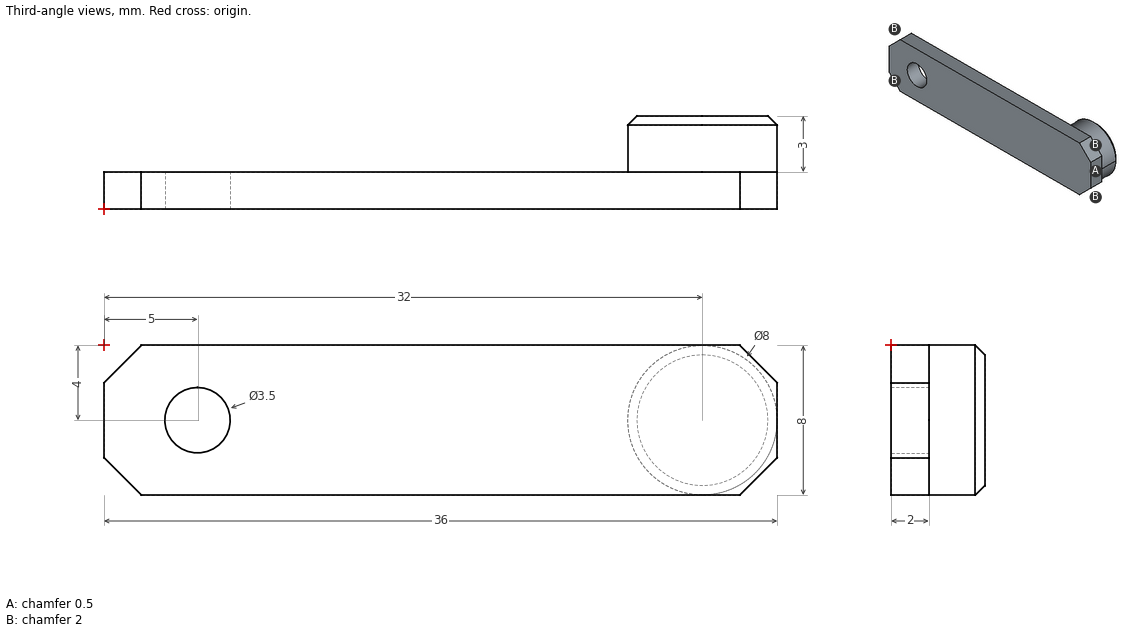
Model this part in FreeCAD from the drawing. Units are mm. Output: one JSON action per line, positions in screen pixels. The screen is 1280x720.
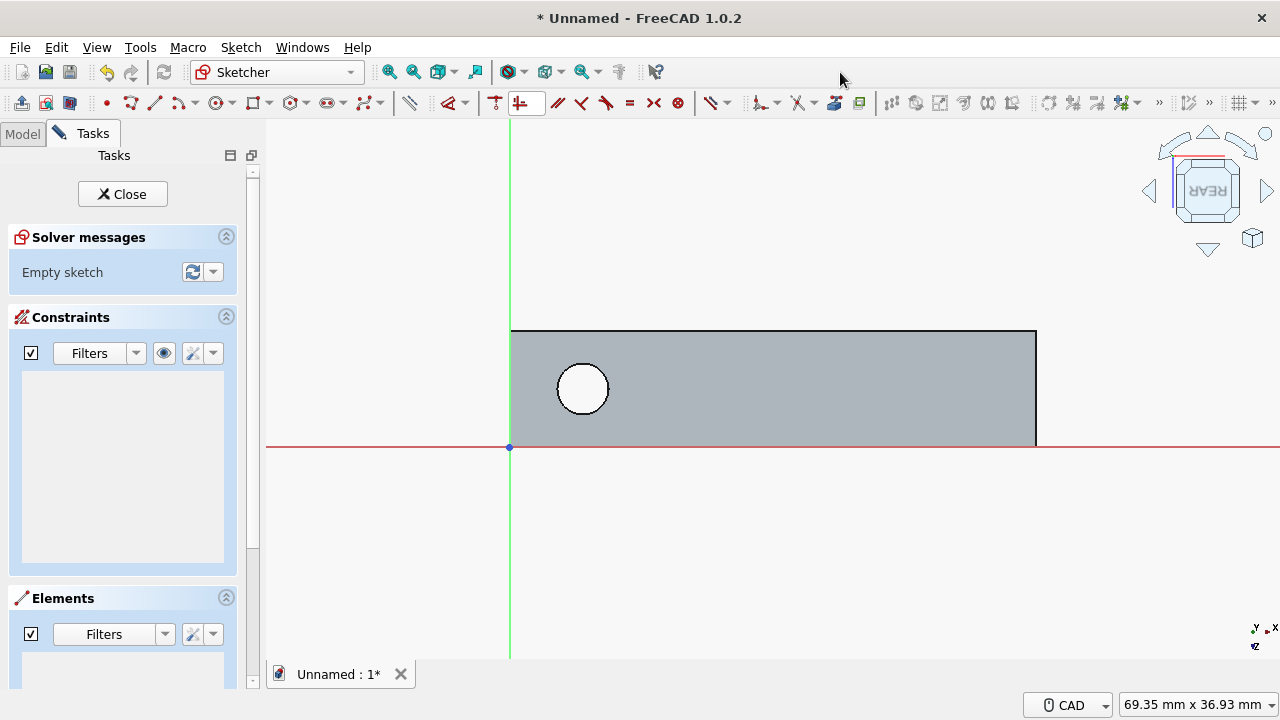
{"action": "scroll", "coordinate": [1115, 389], "scroll_direction": "up", "scroll_amount": 5}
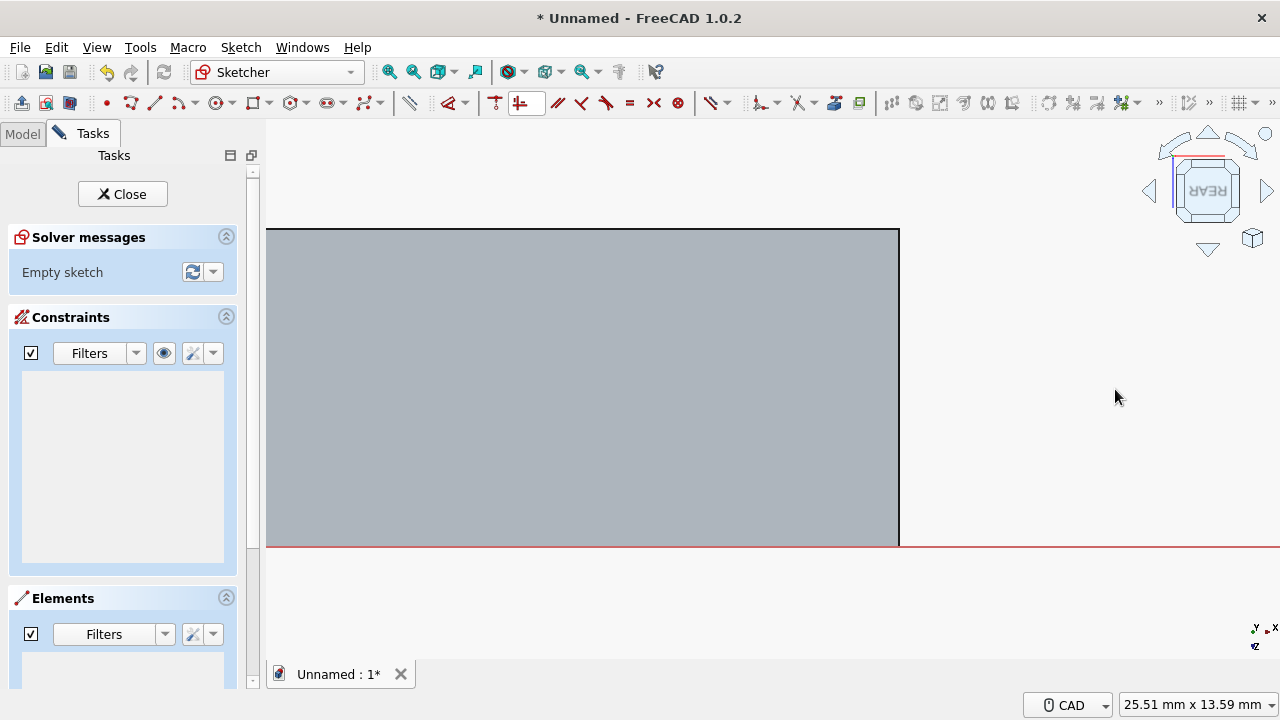
{"action": "key", "text": "g c"}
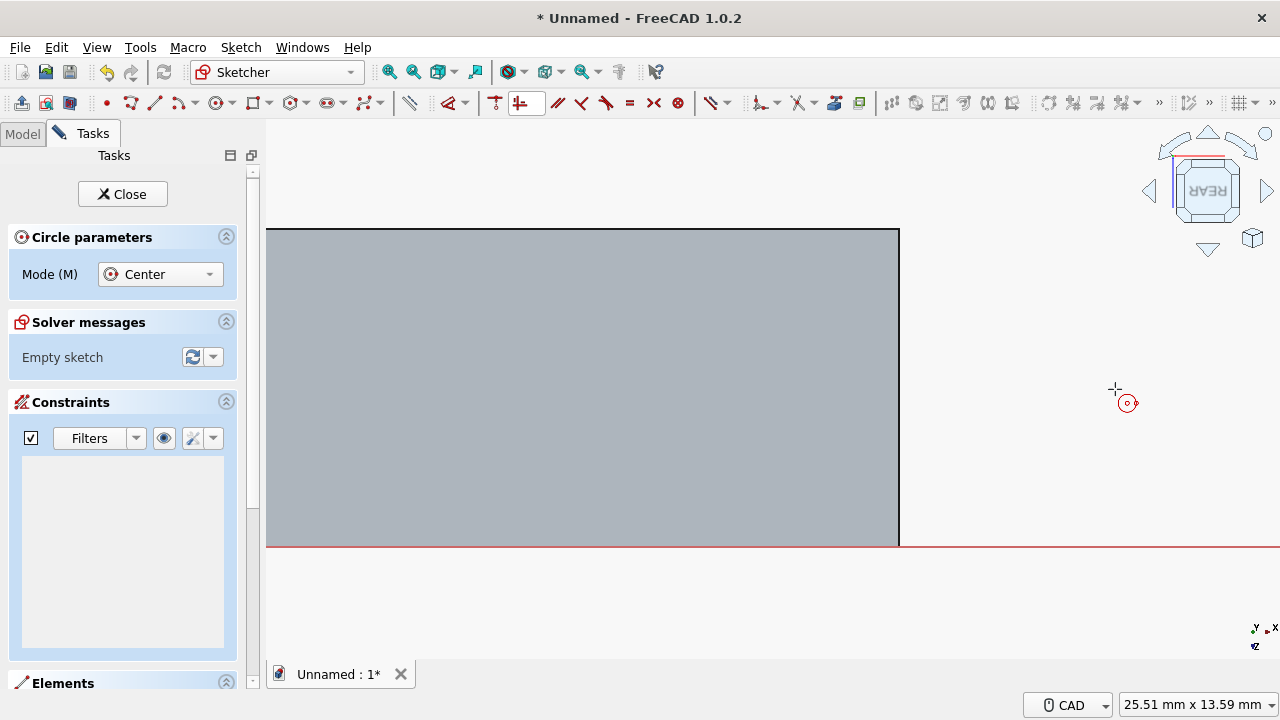
{"action": "left_click", "coordinate": [740, 388]}
{"action": "mouse_move", "coordinate": [853, 276]}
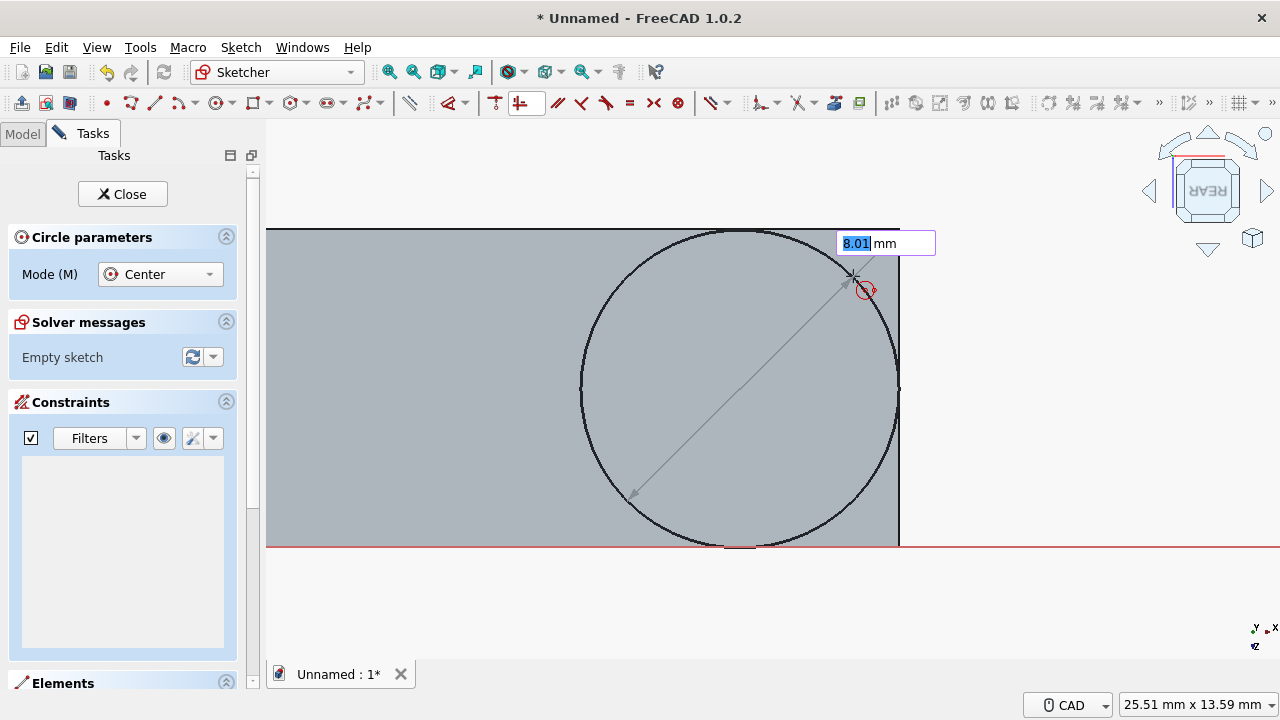
{"action": "type", "text": "8"}
{"action": "key", "text": "Return"}
{"action": "key", "text": "Escape"}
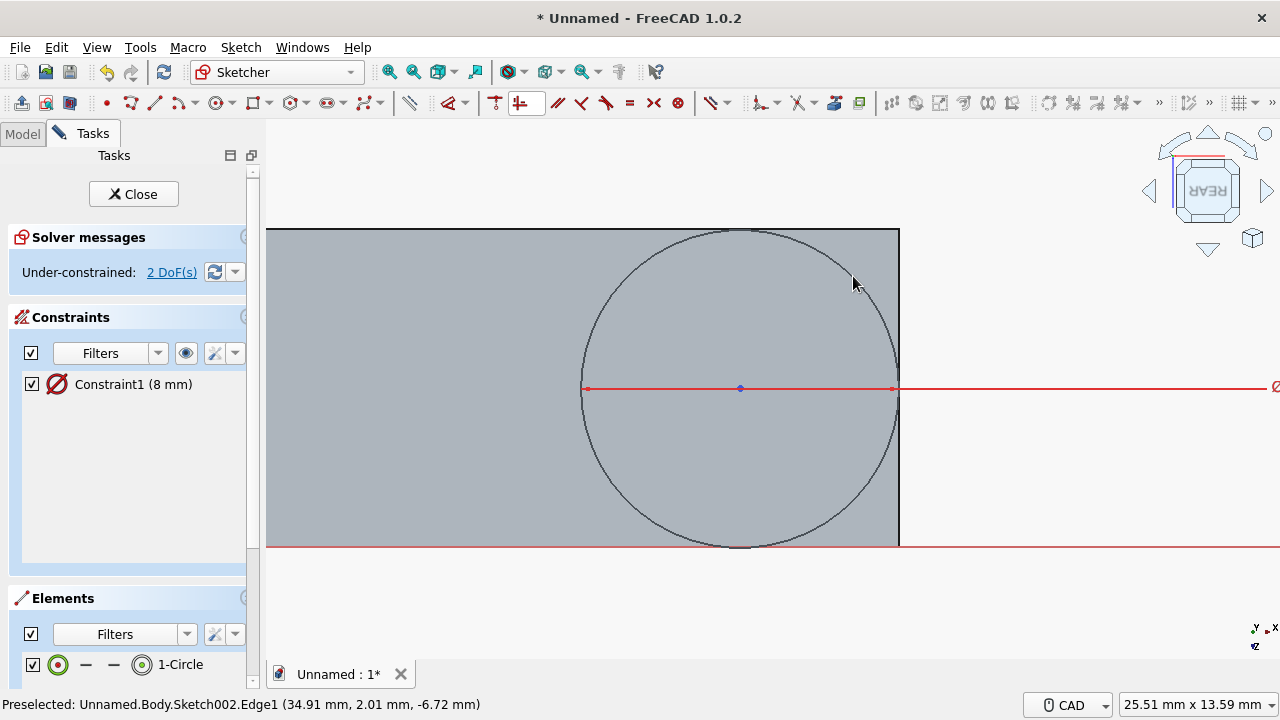
{"action": "key", "text": "d"}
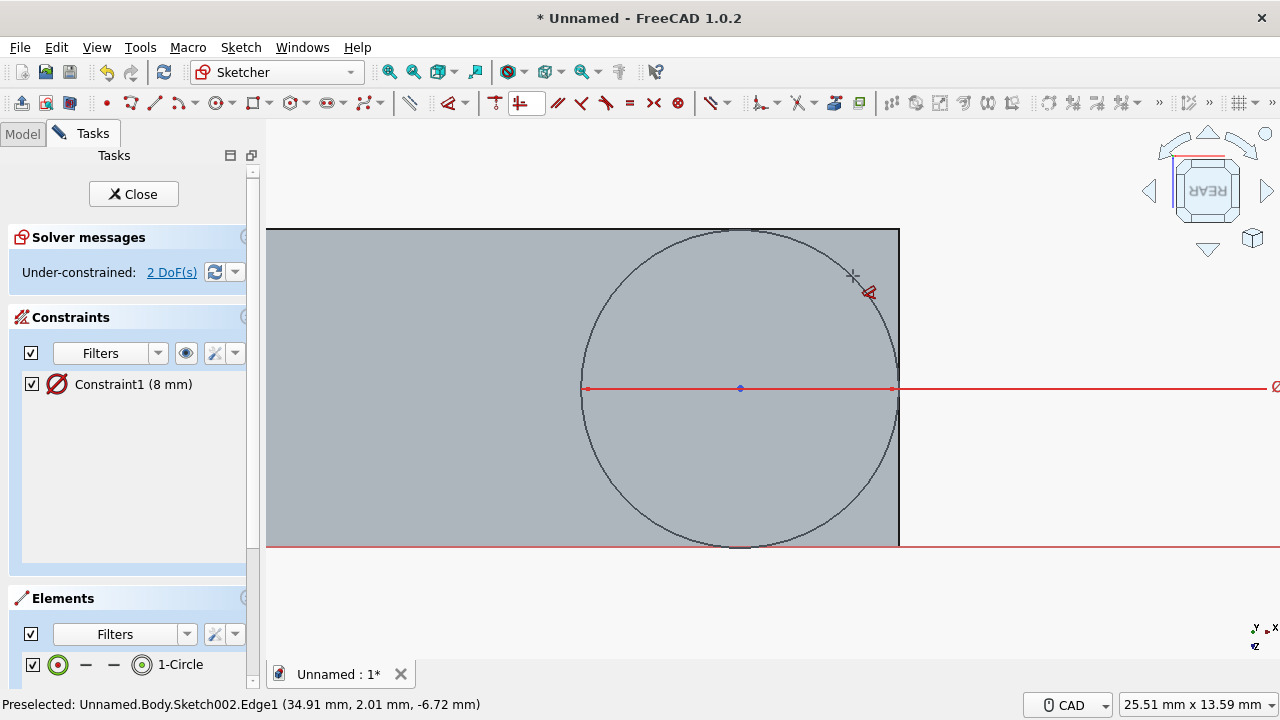
{"action": "left_click", "coordinate": [740, 389]}
{"action": "left_click", "coordinate": [774, 468]}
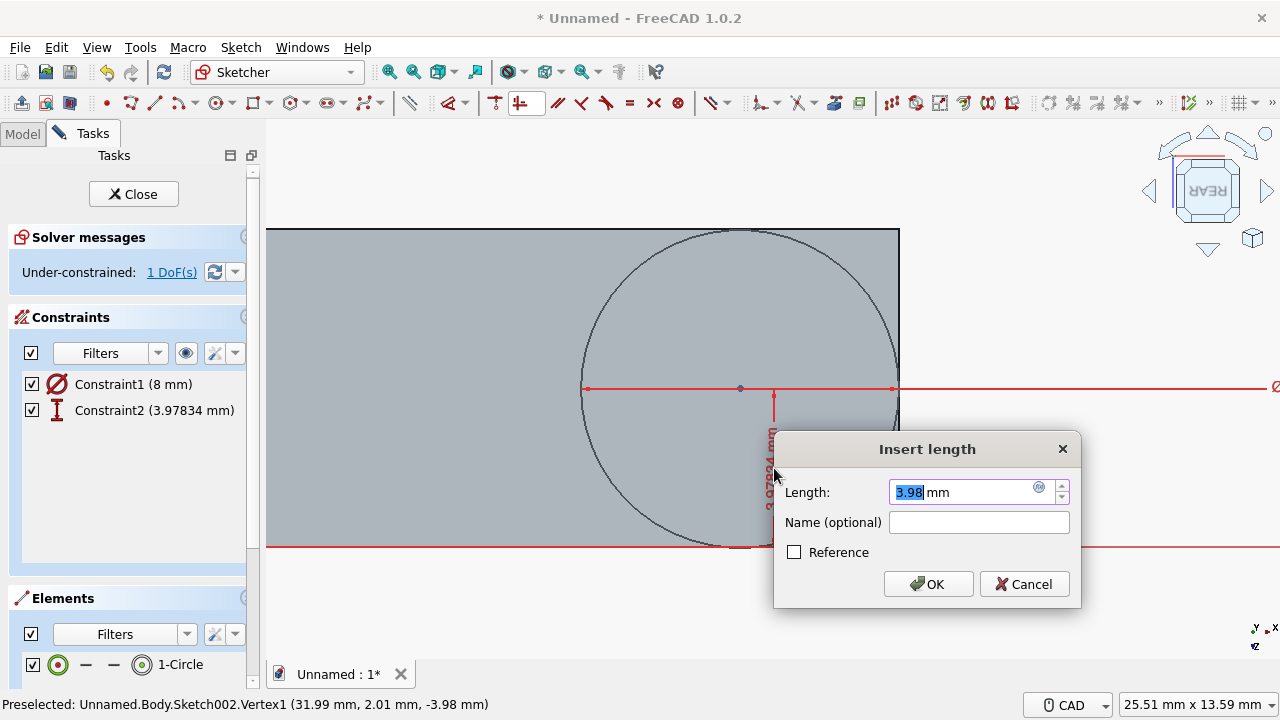
{"action": "type", "text": "4"}
{"action": "key", "text": "Return"}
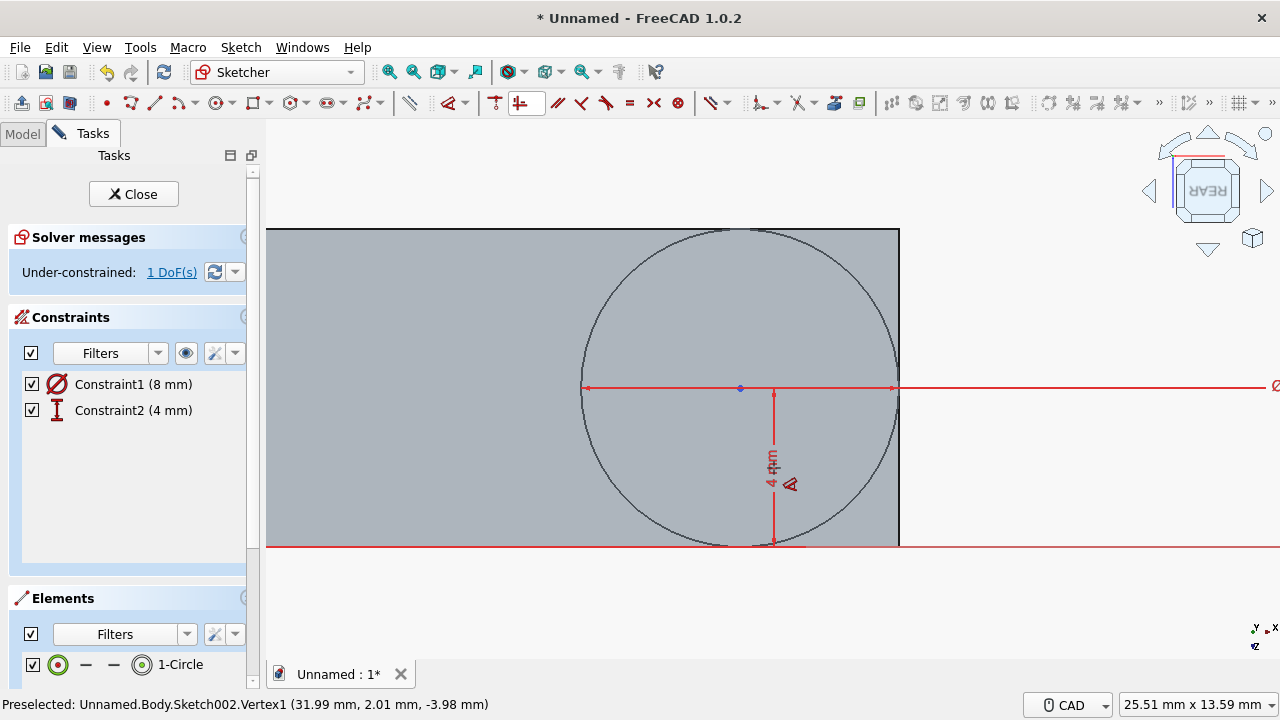
{"action": "left_click", "coordinate": [740, 388]}
{"action": "left_click", "coordinate": [517, 581]}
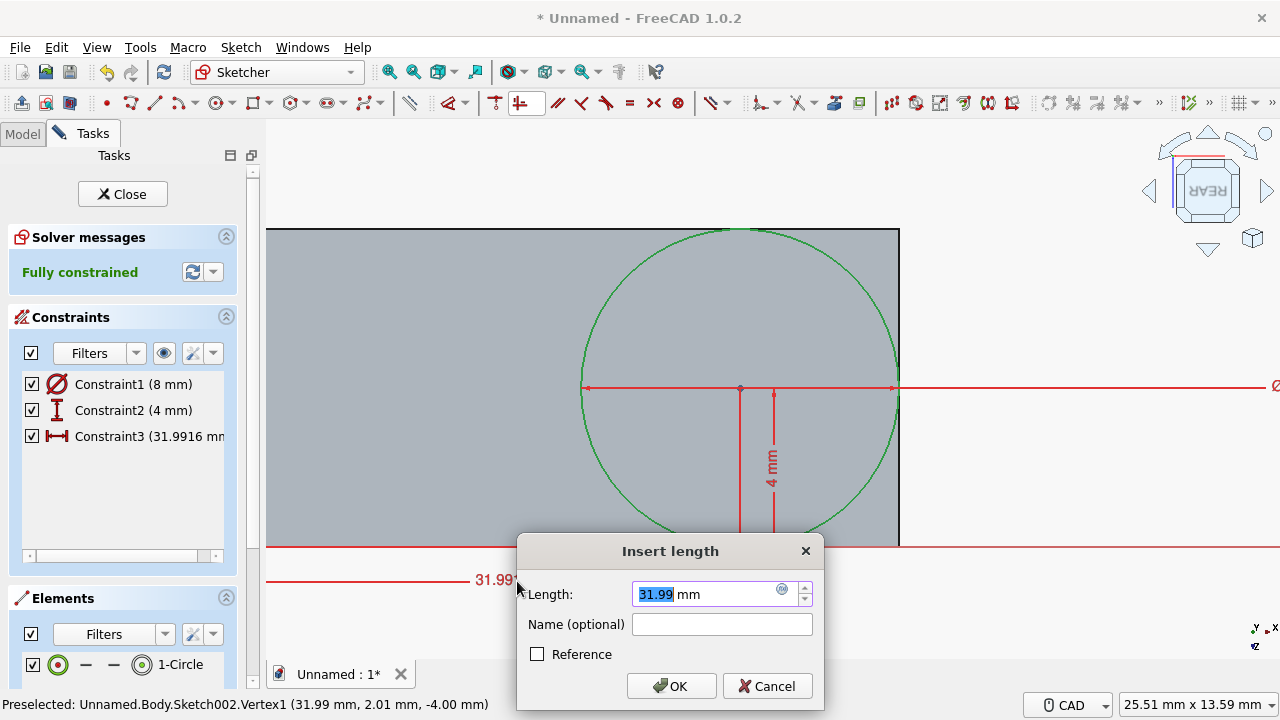
{"action": "type", "text": "32"}
{"action": "key", "text": "Return"}
{"action": "key", "text": "Escape"}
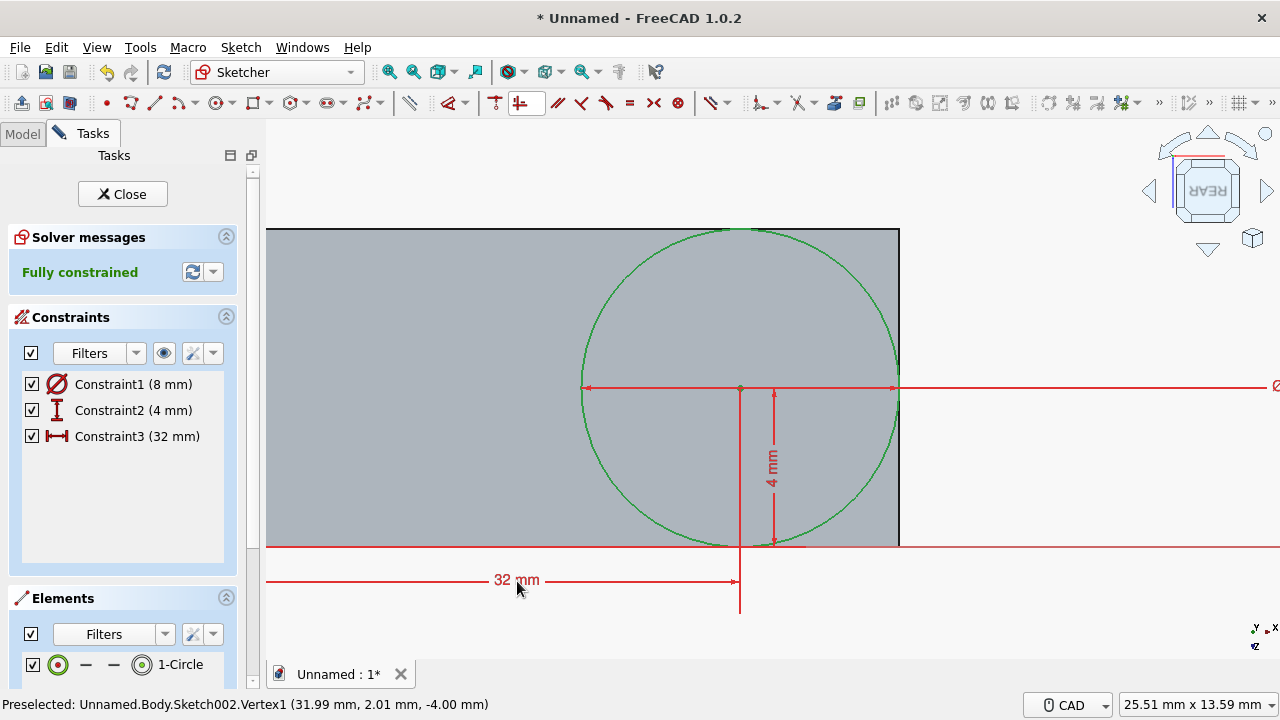
{"action": "left_click", "coordinate": [123, 194]}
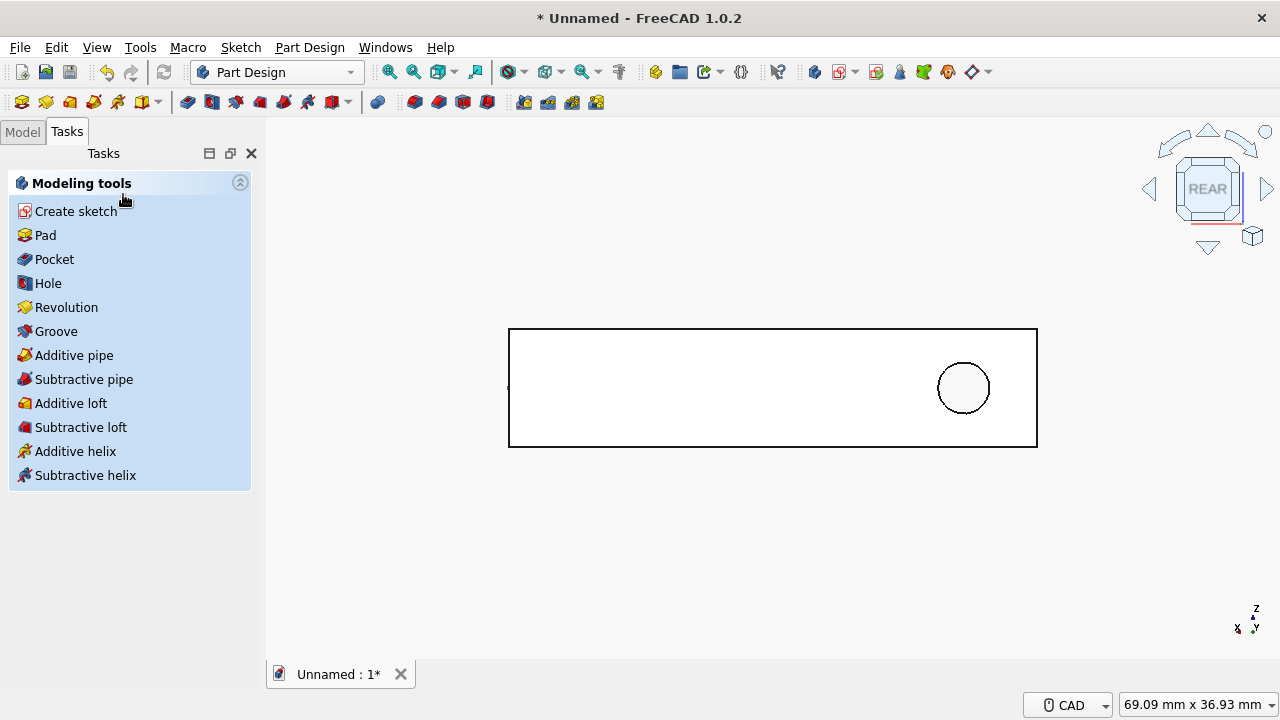
{"action": "left_click", "coordinate": [22, 102]}